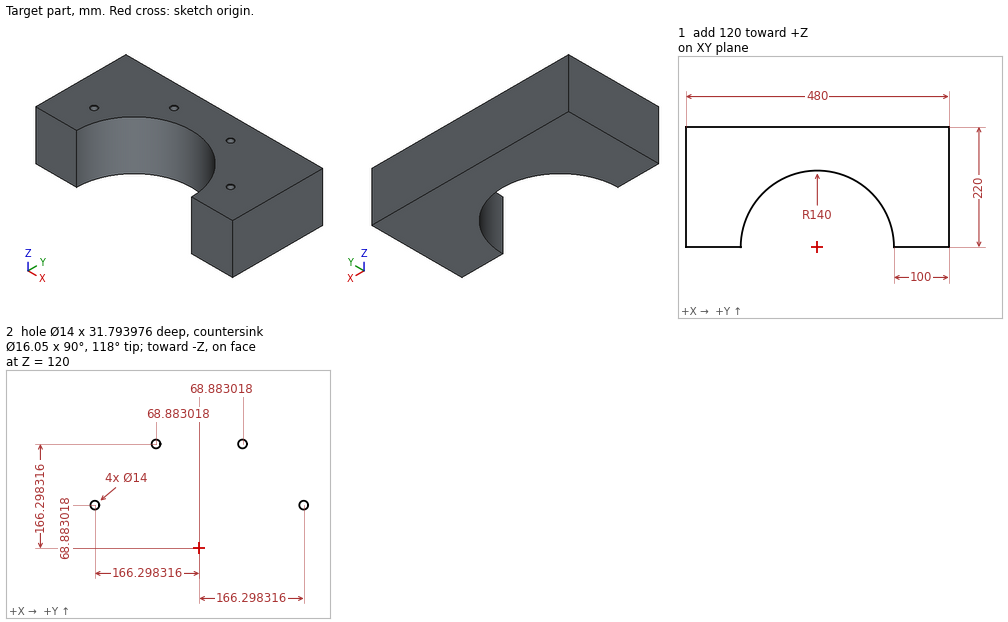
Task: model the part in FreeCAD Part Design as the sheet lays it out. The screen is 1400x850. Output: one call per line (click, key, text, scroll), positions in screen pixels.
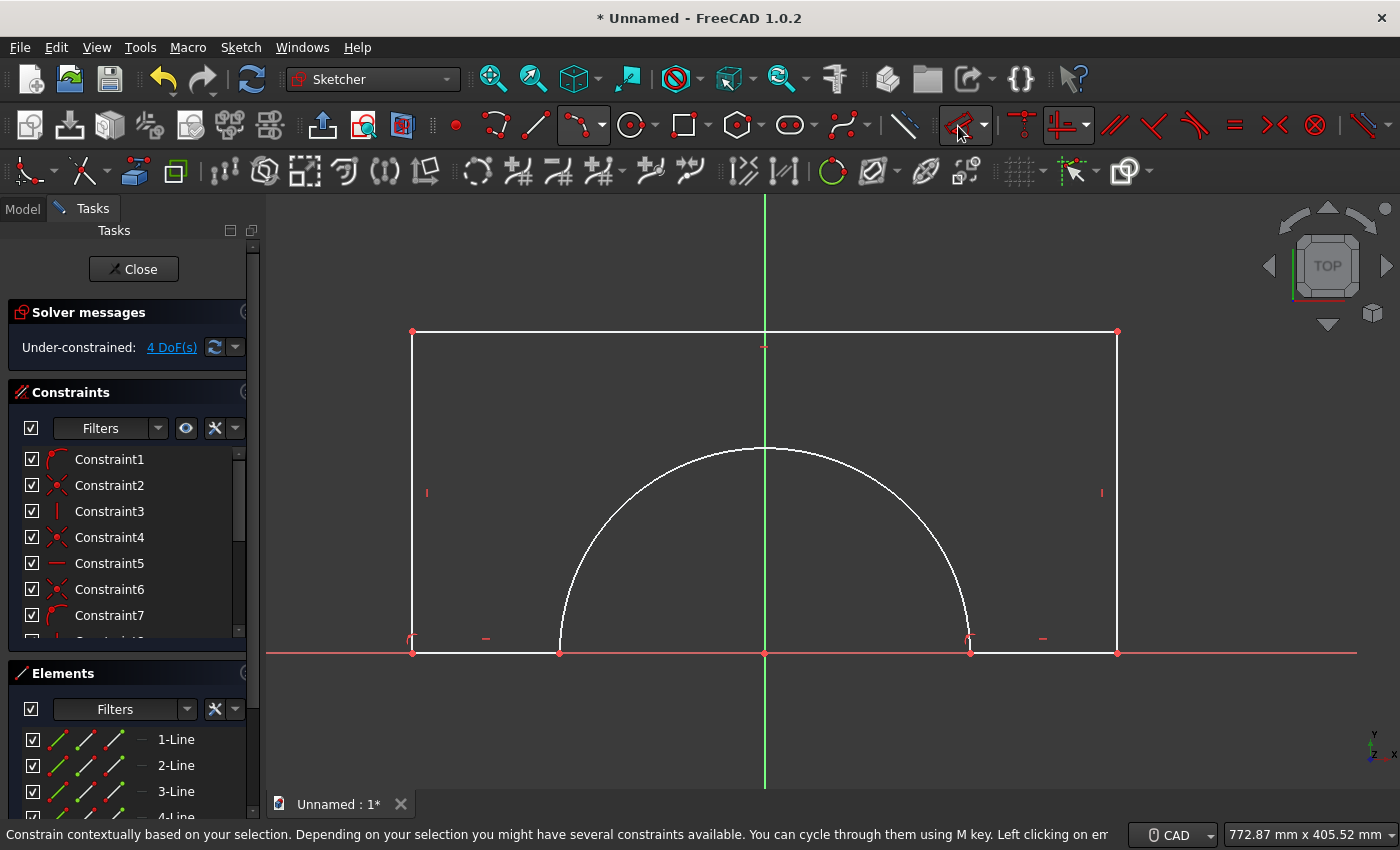
click(886, 487)
click(905, 461)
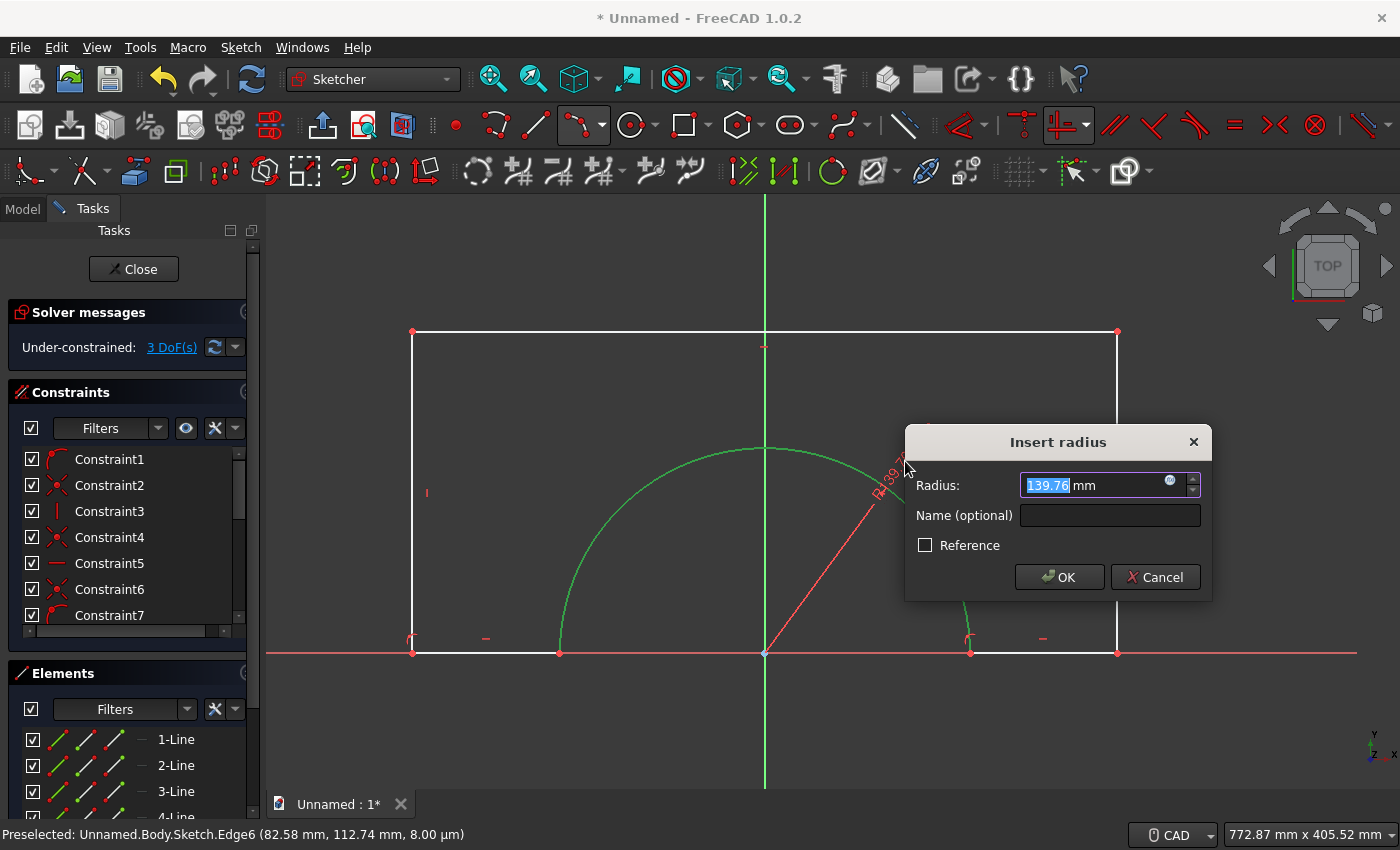
text(140)
key(Return)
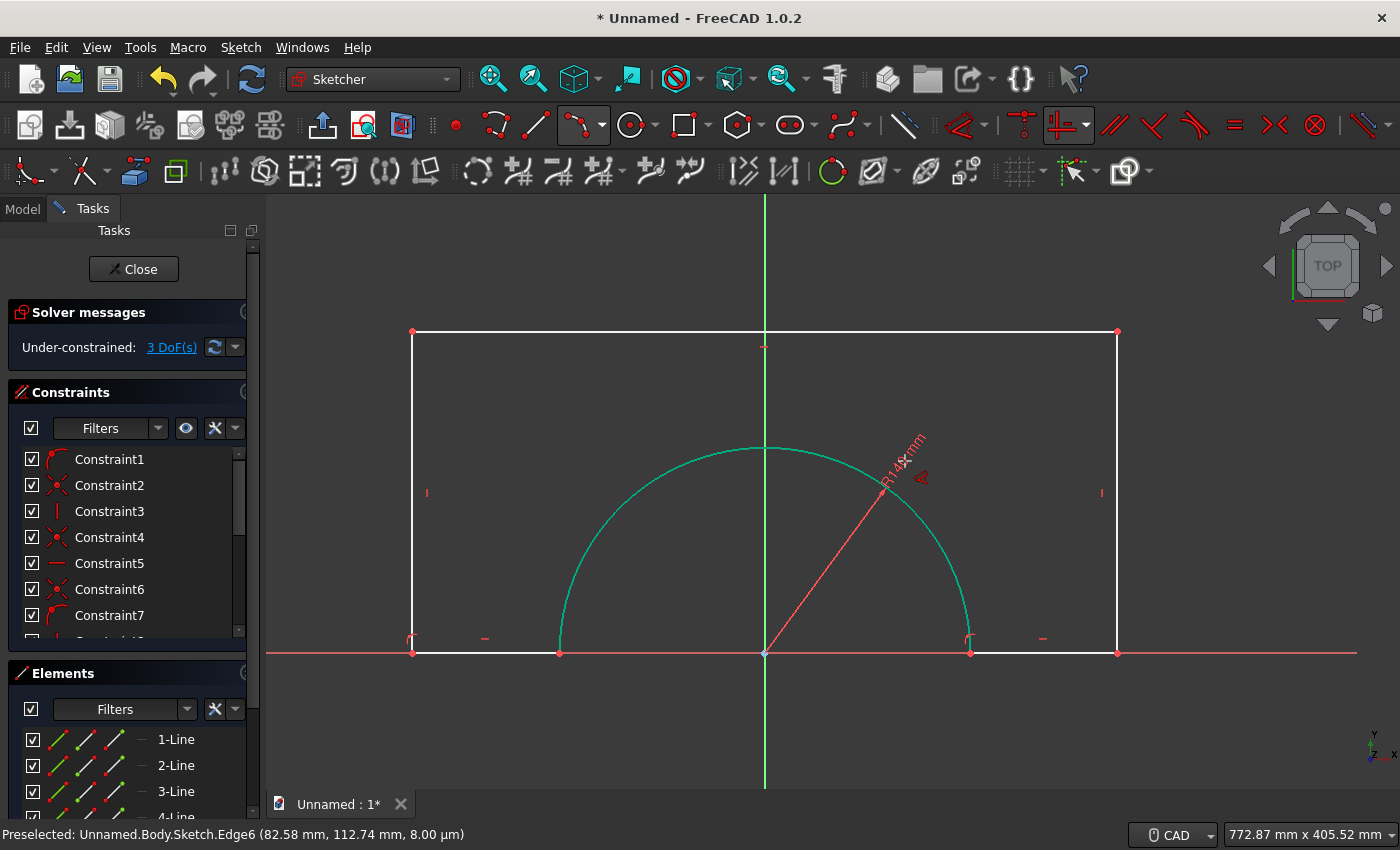
click(1014, 653)
click(1044, 687)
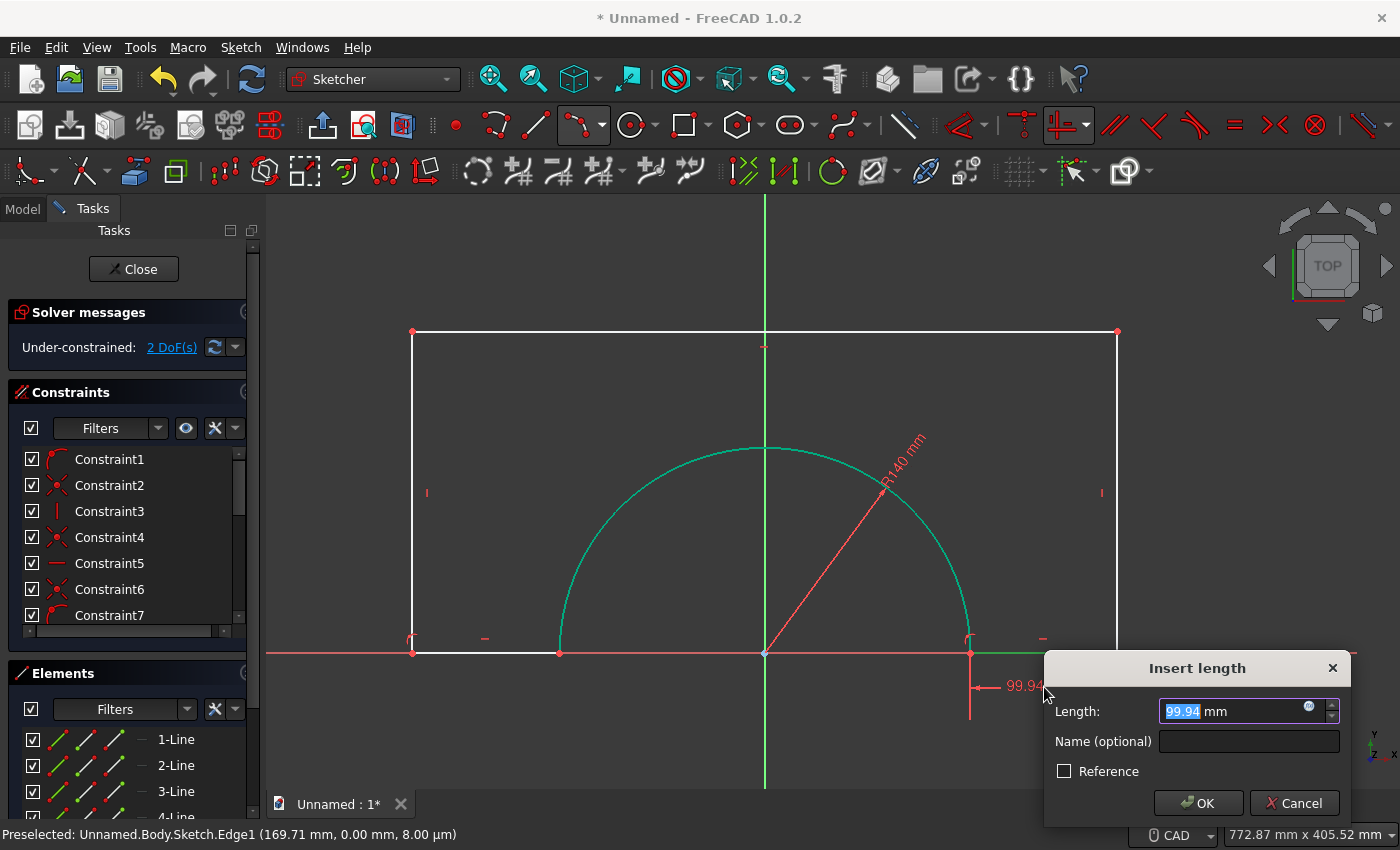
text(100)
key(Return)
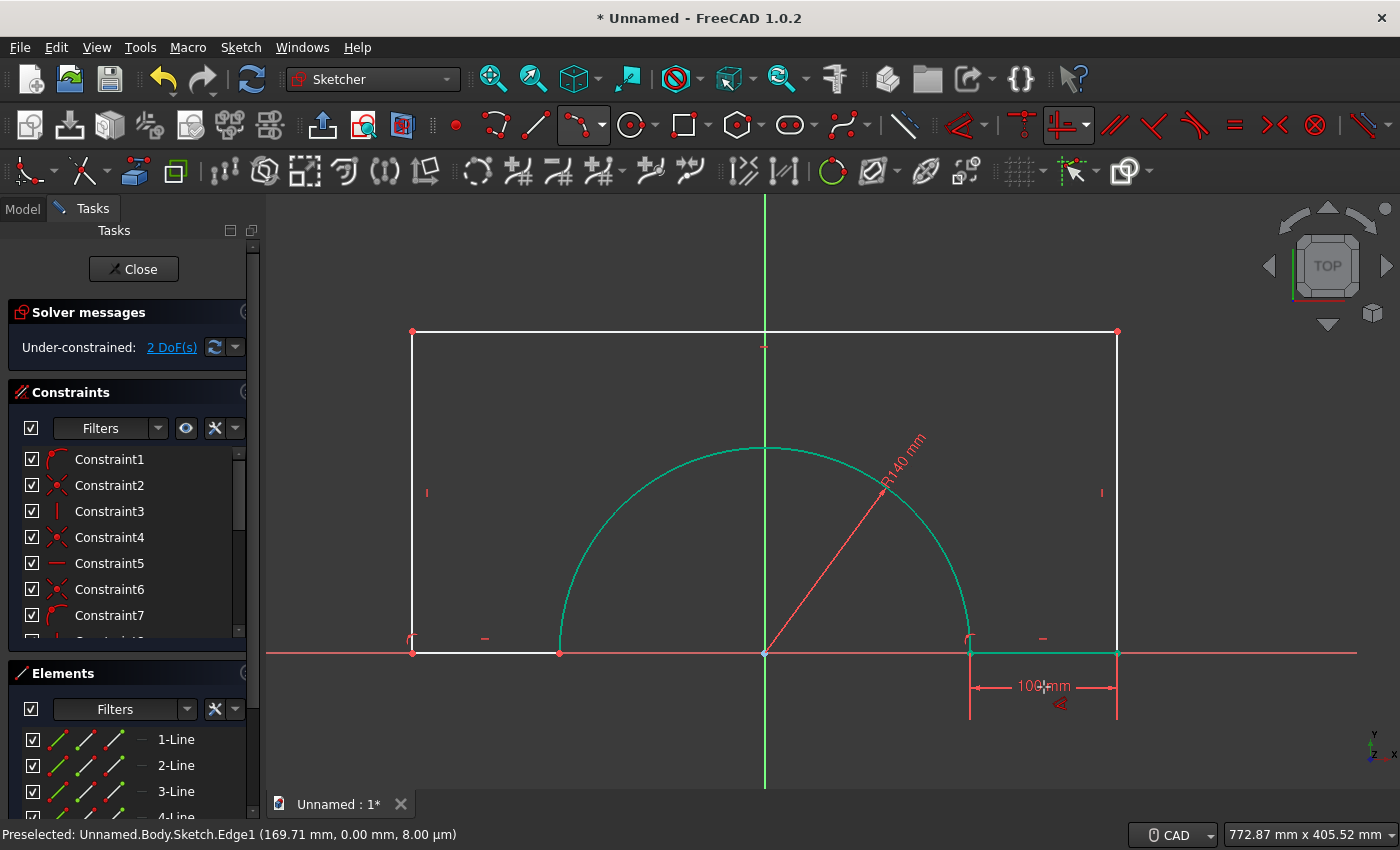
click(1117, 557)
click(1151, 492)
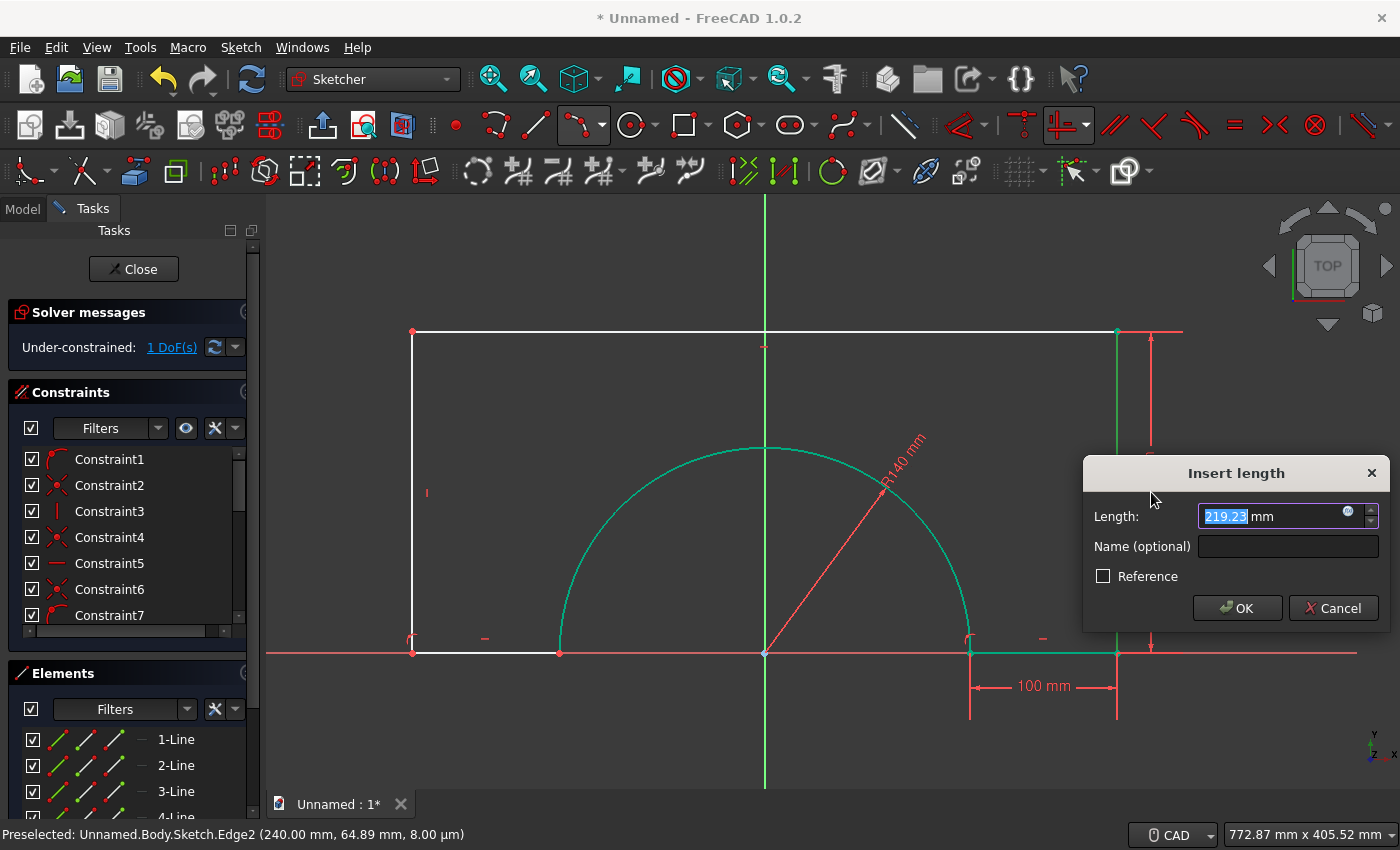
text(220)
key(Return)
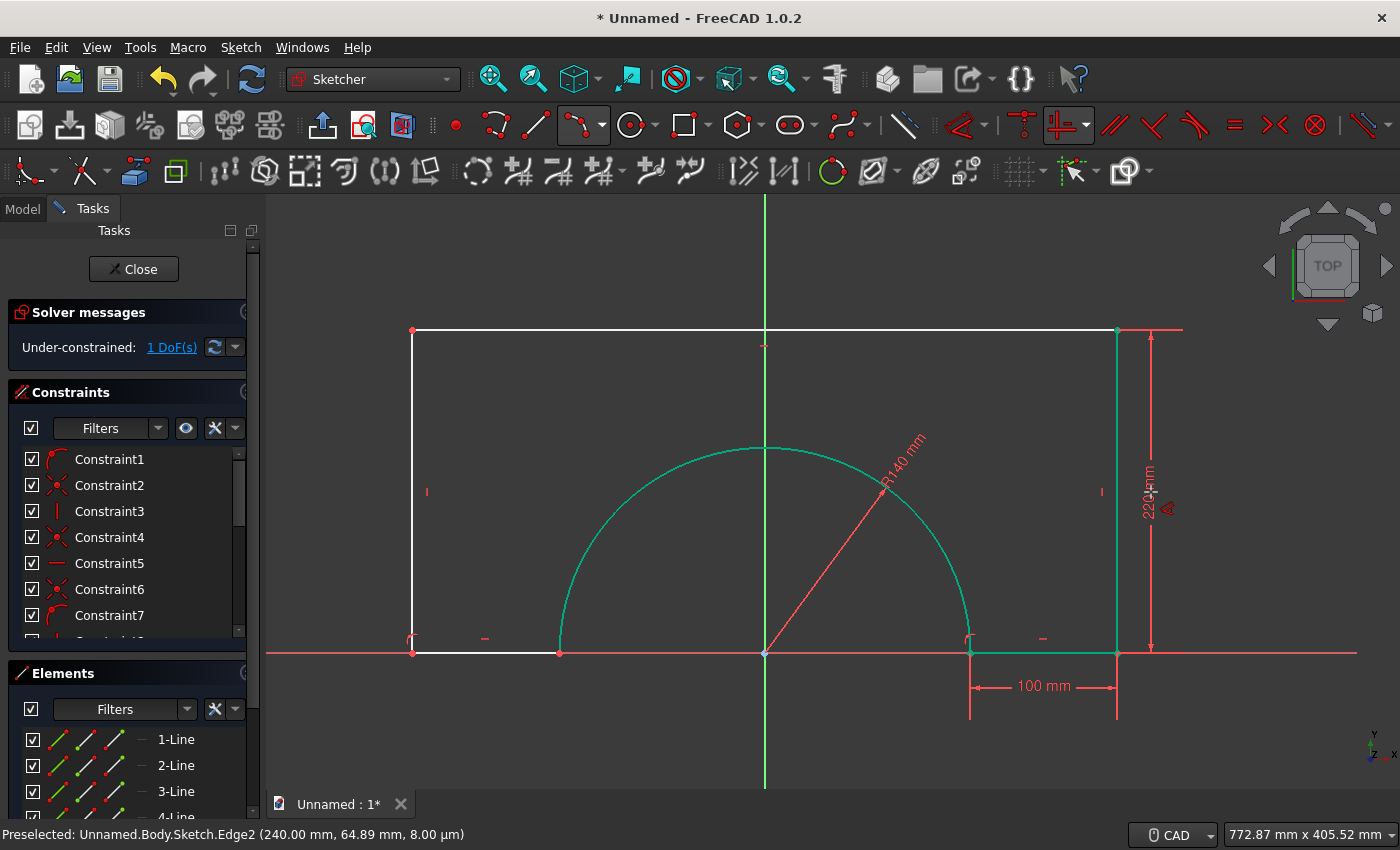
click(906, 330)
click(603, 296)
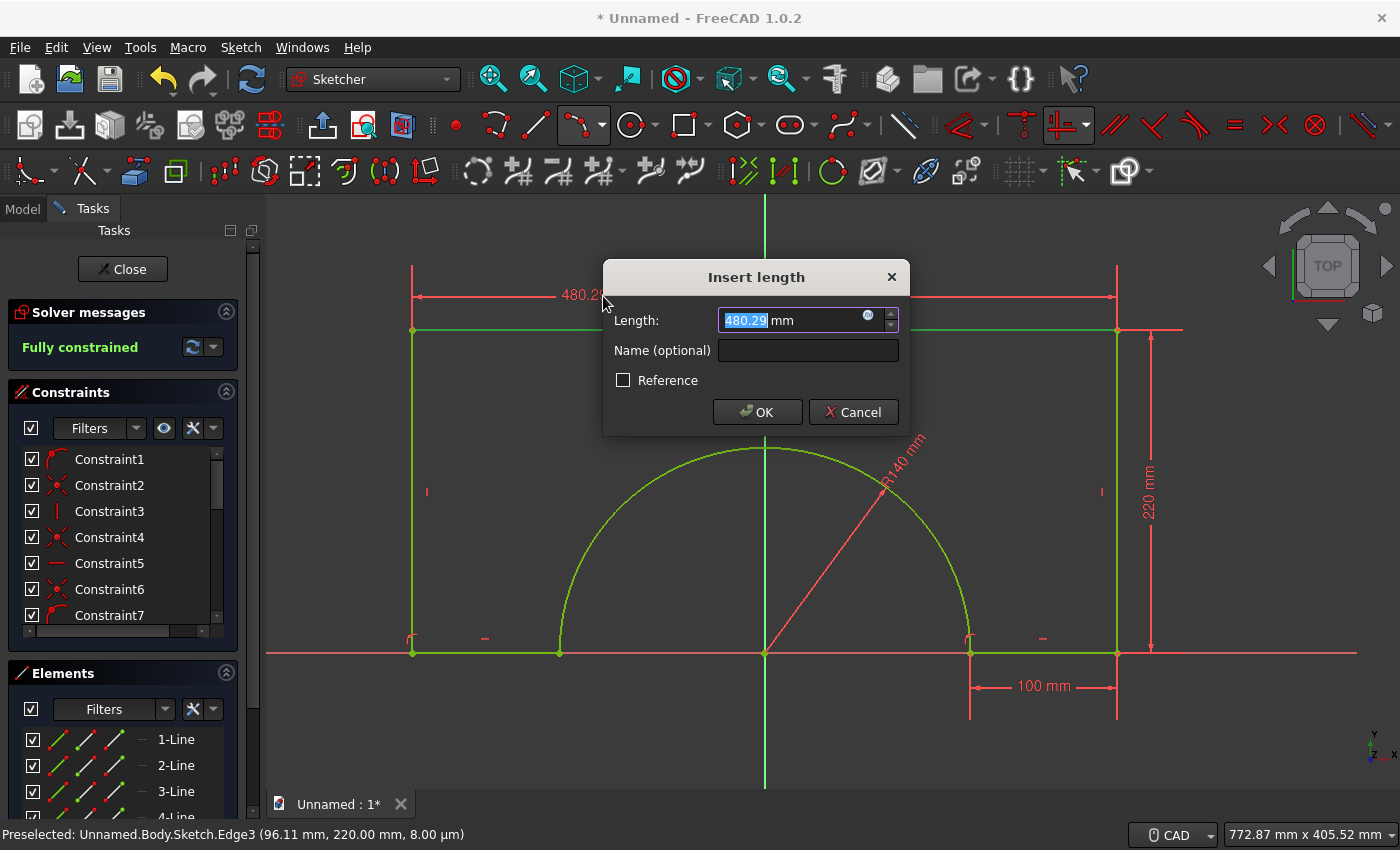
text(480)
key(Return)
key(Escape)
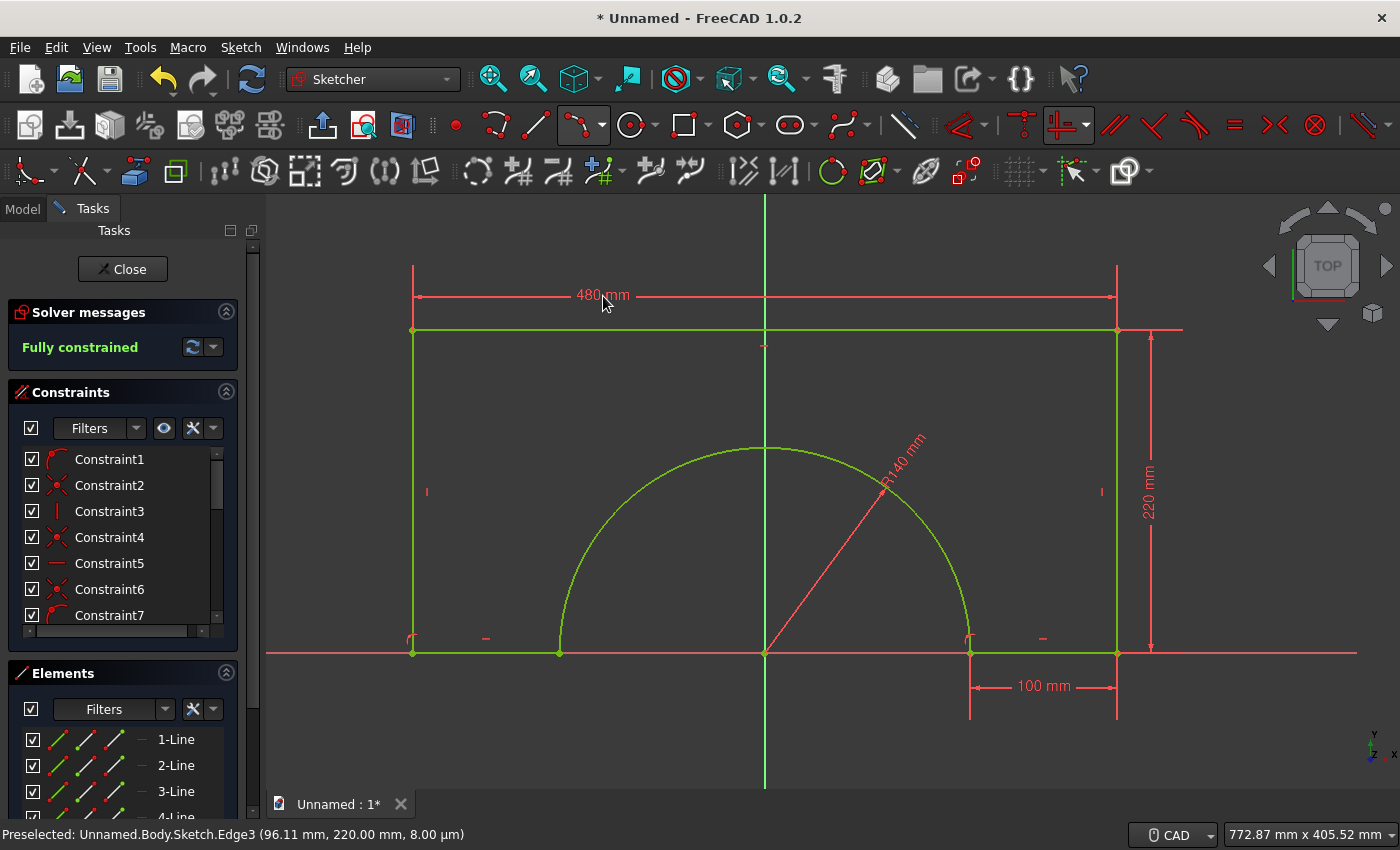
click(123, 269)